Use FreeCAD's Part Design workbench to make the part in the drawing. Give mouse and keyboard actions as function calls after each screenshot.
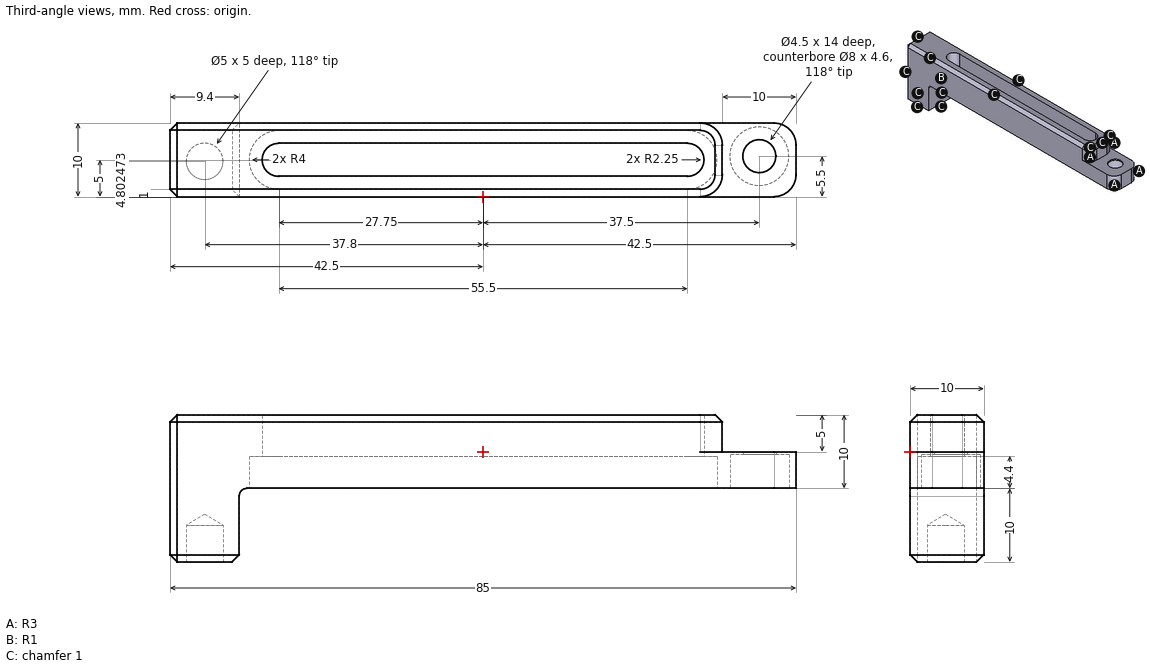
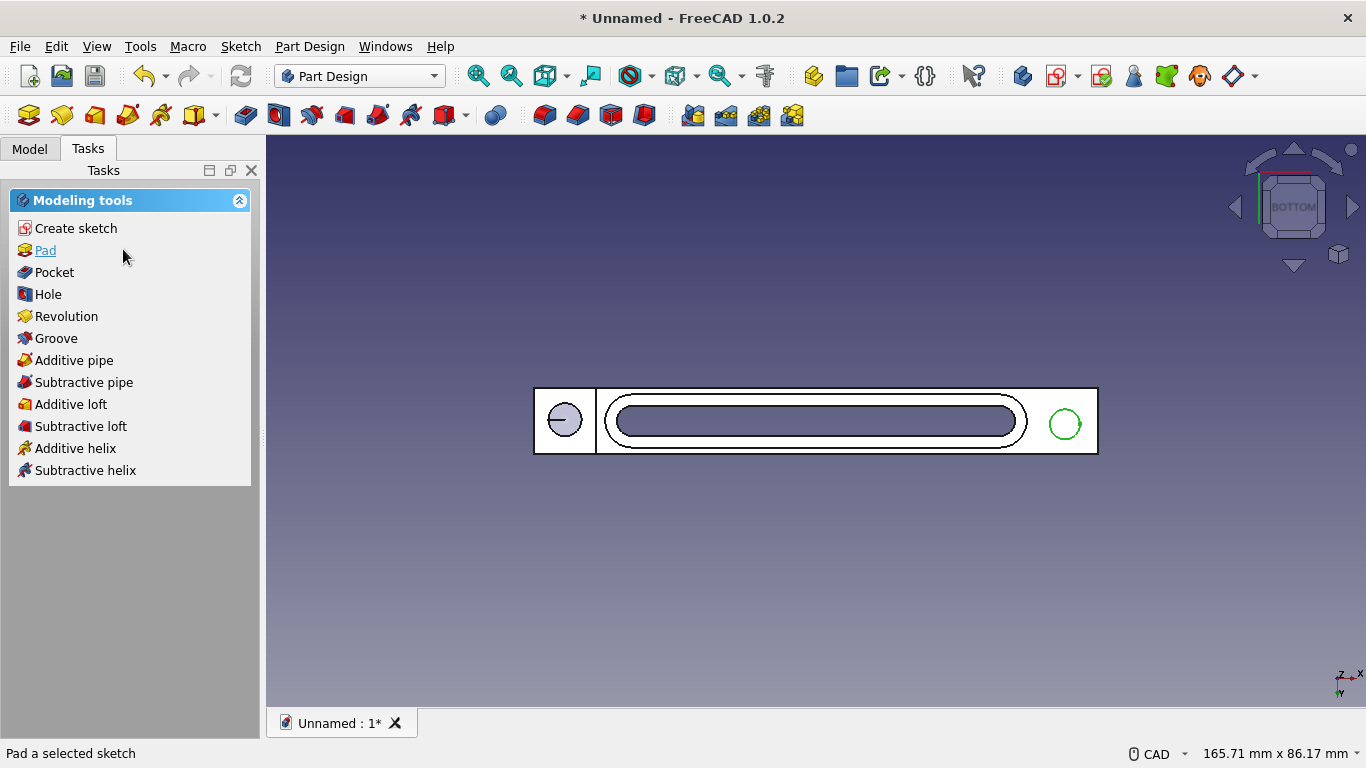
click(279, 116)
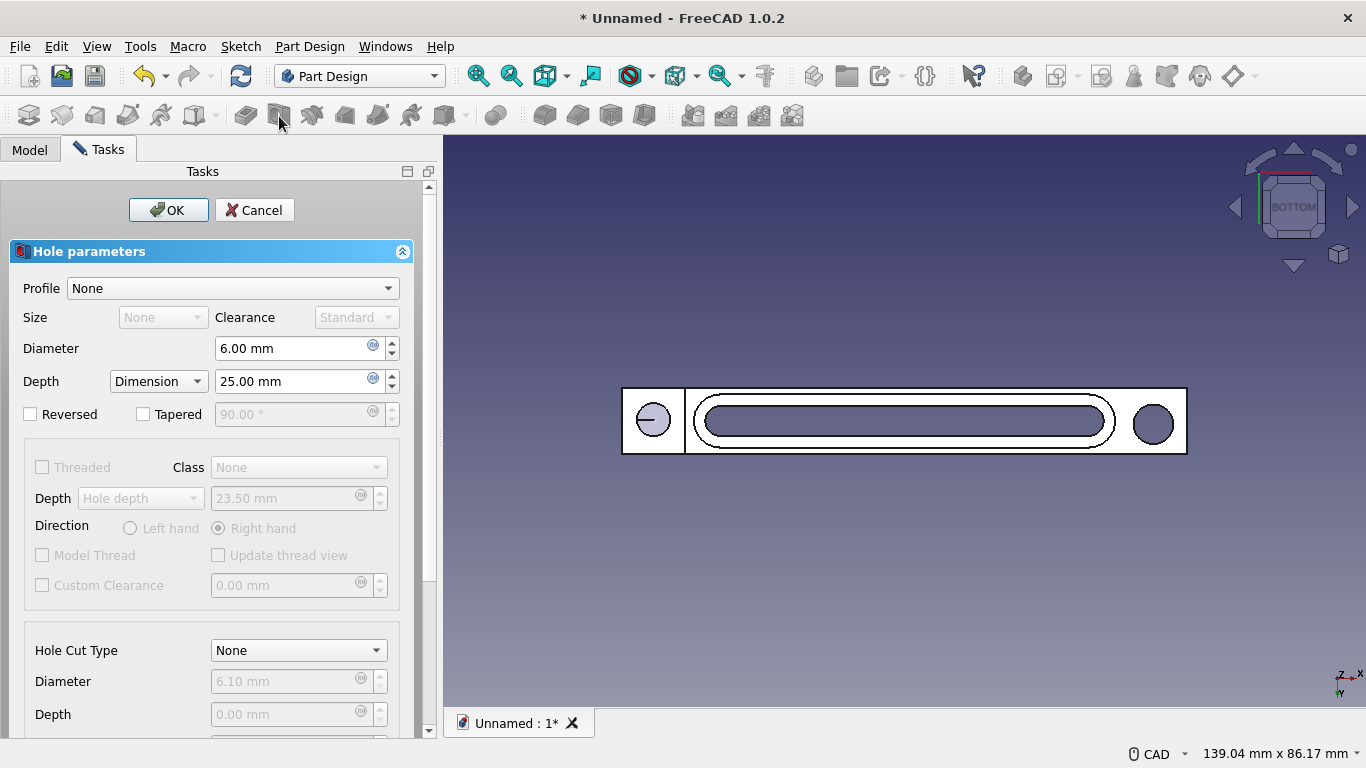
triple_click(300, 348)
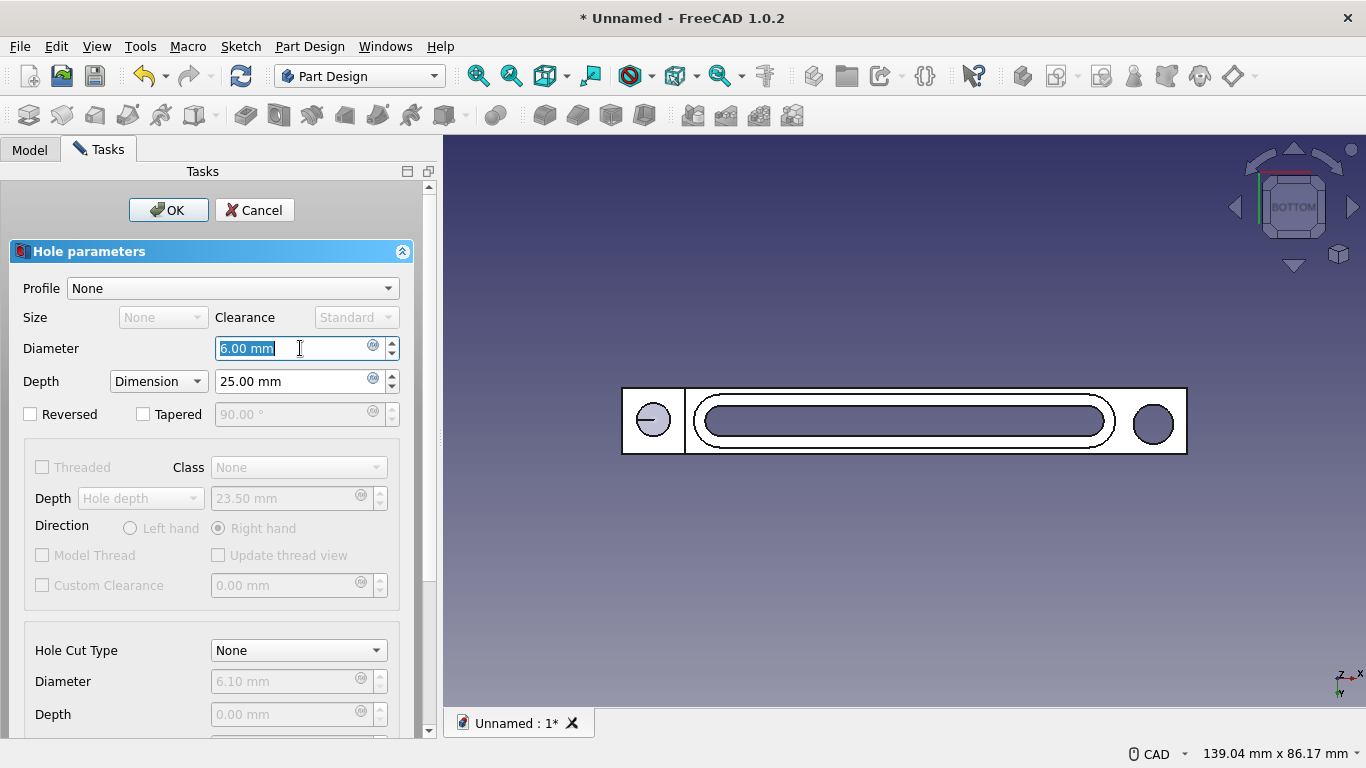
text(4.5)
key(Tab)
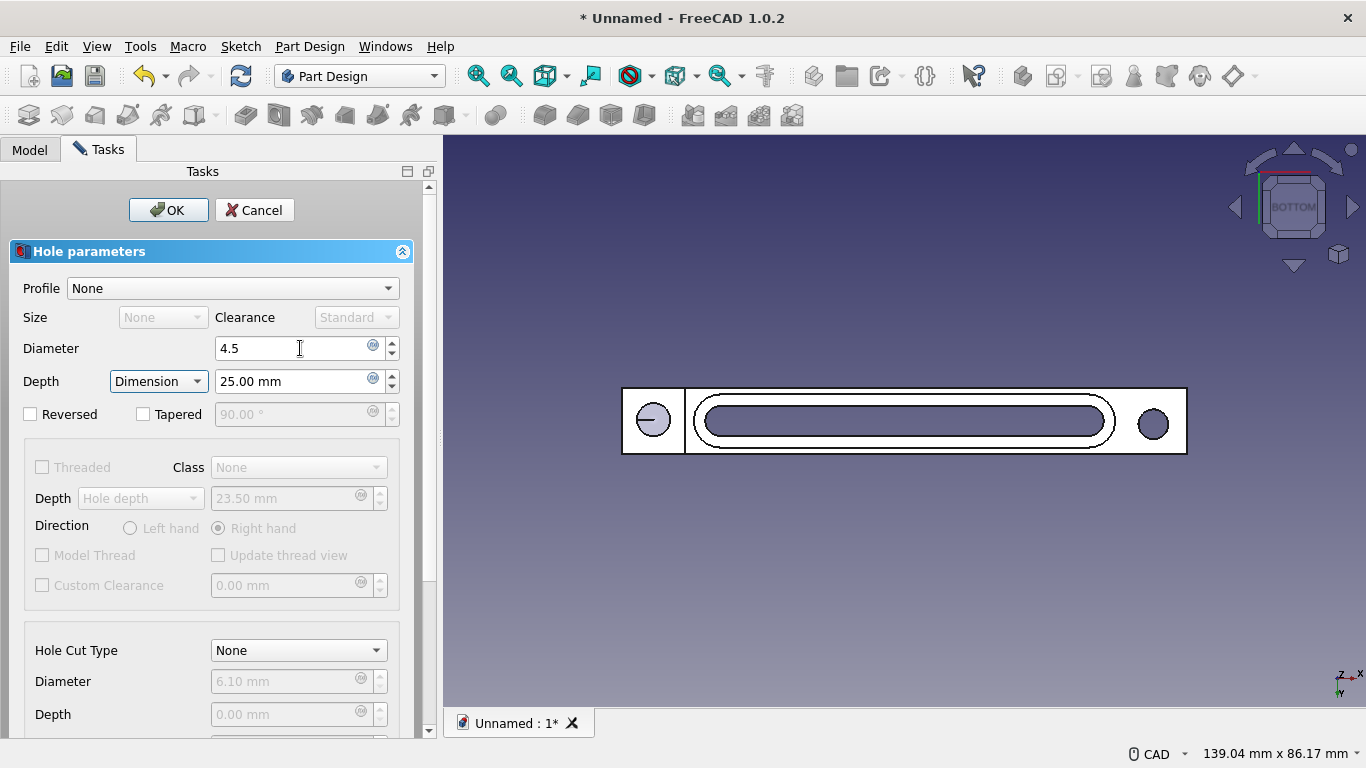
triple_click(300, 382)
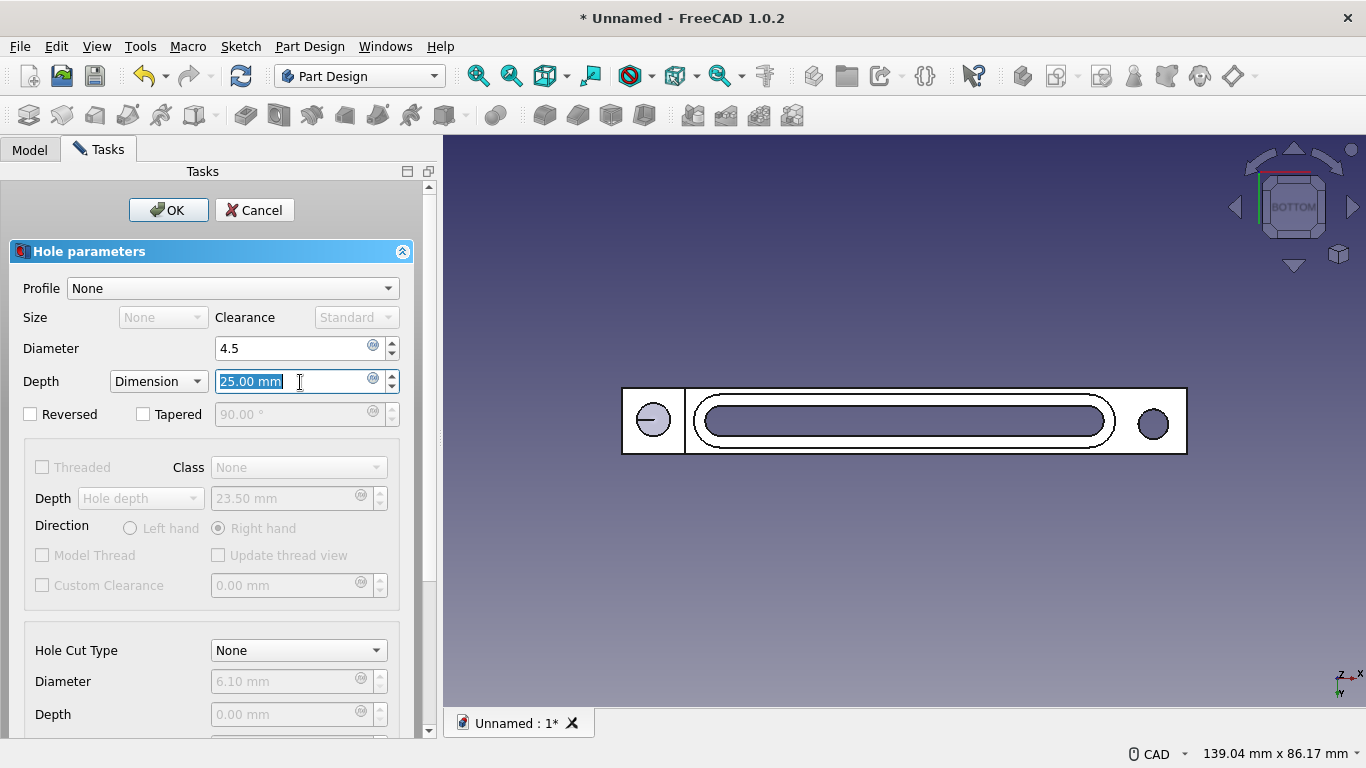
text(14)
key(Tab)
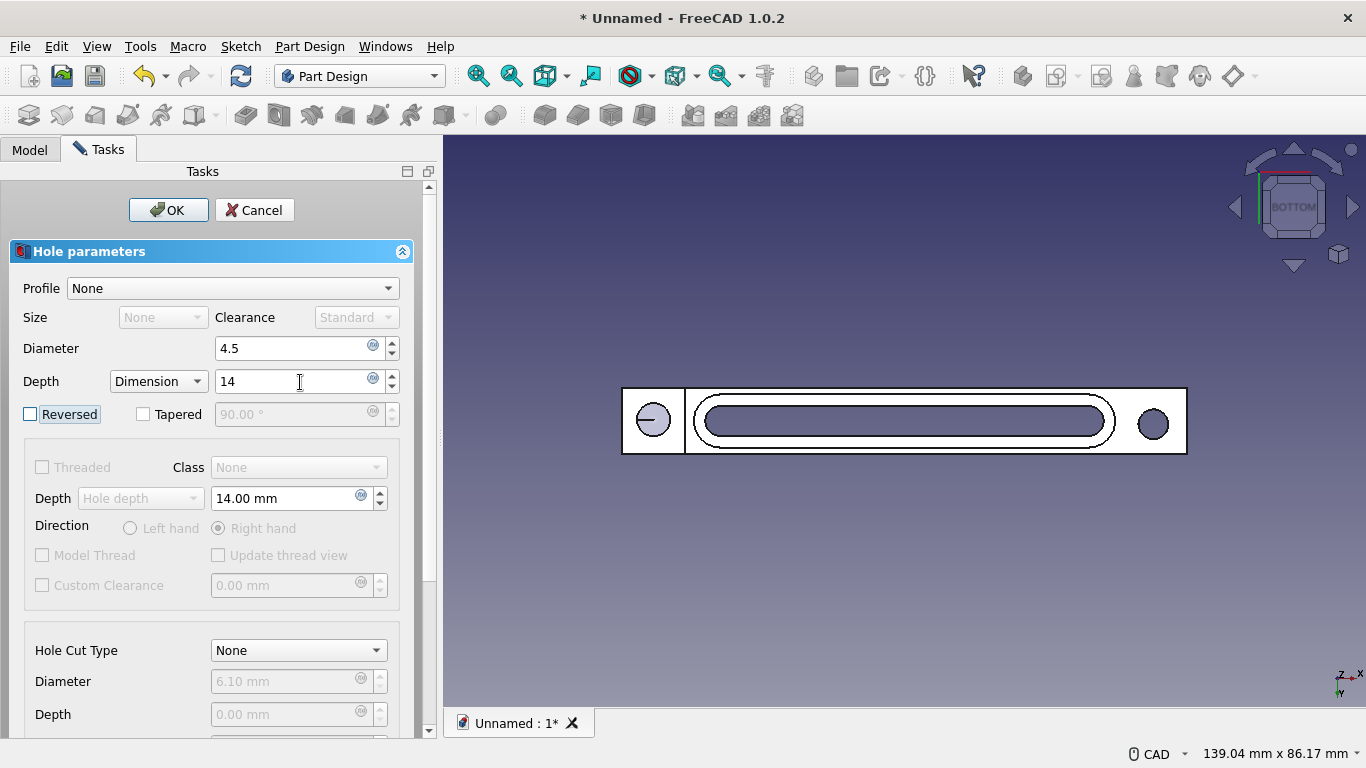
click(300, 650)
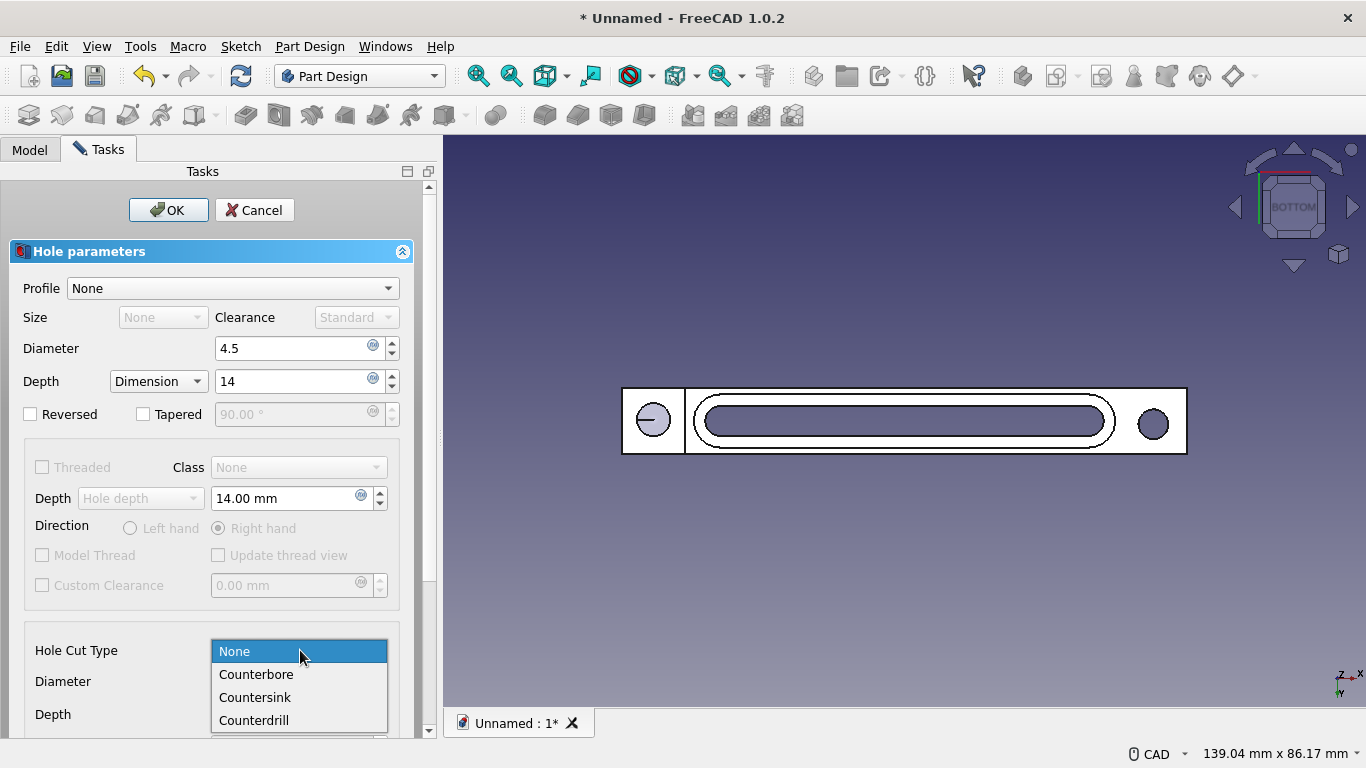
click(298, 674)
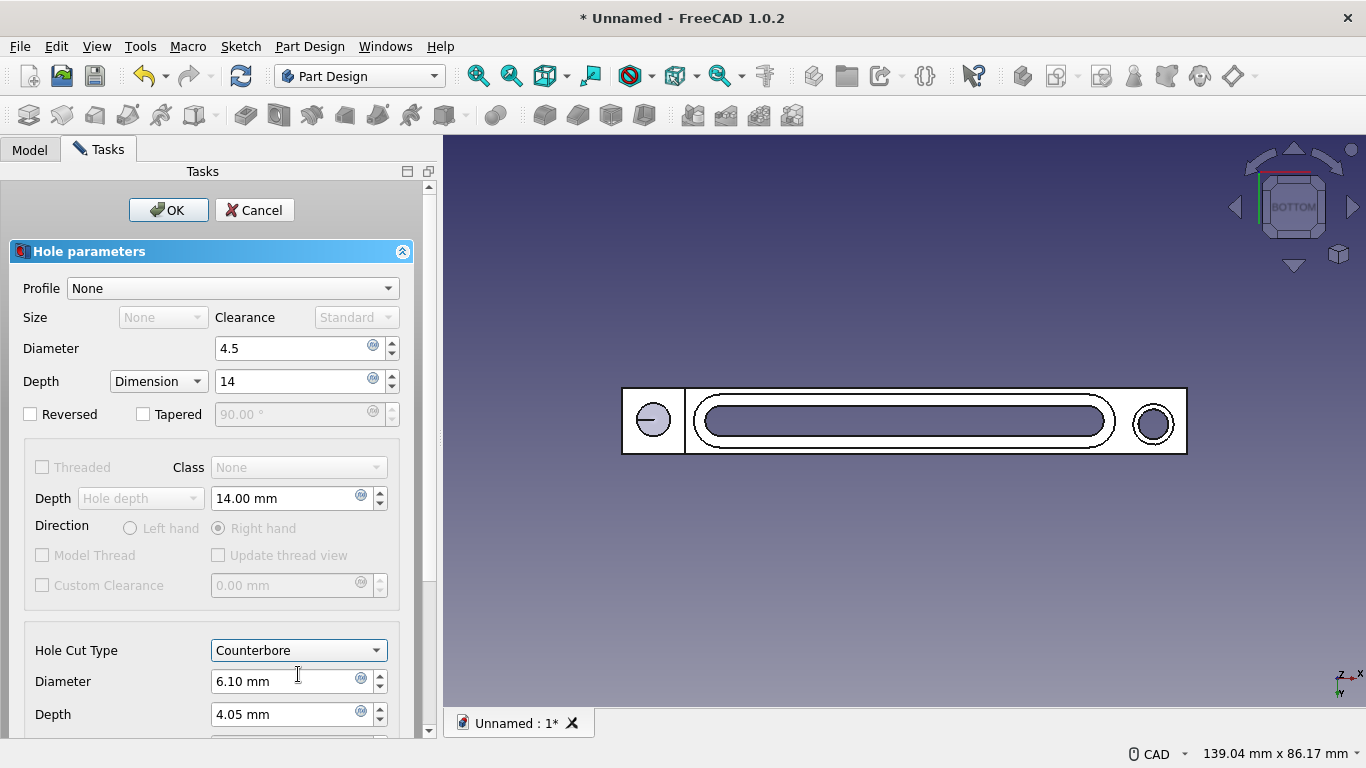
triple_click(292, 682)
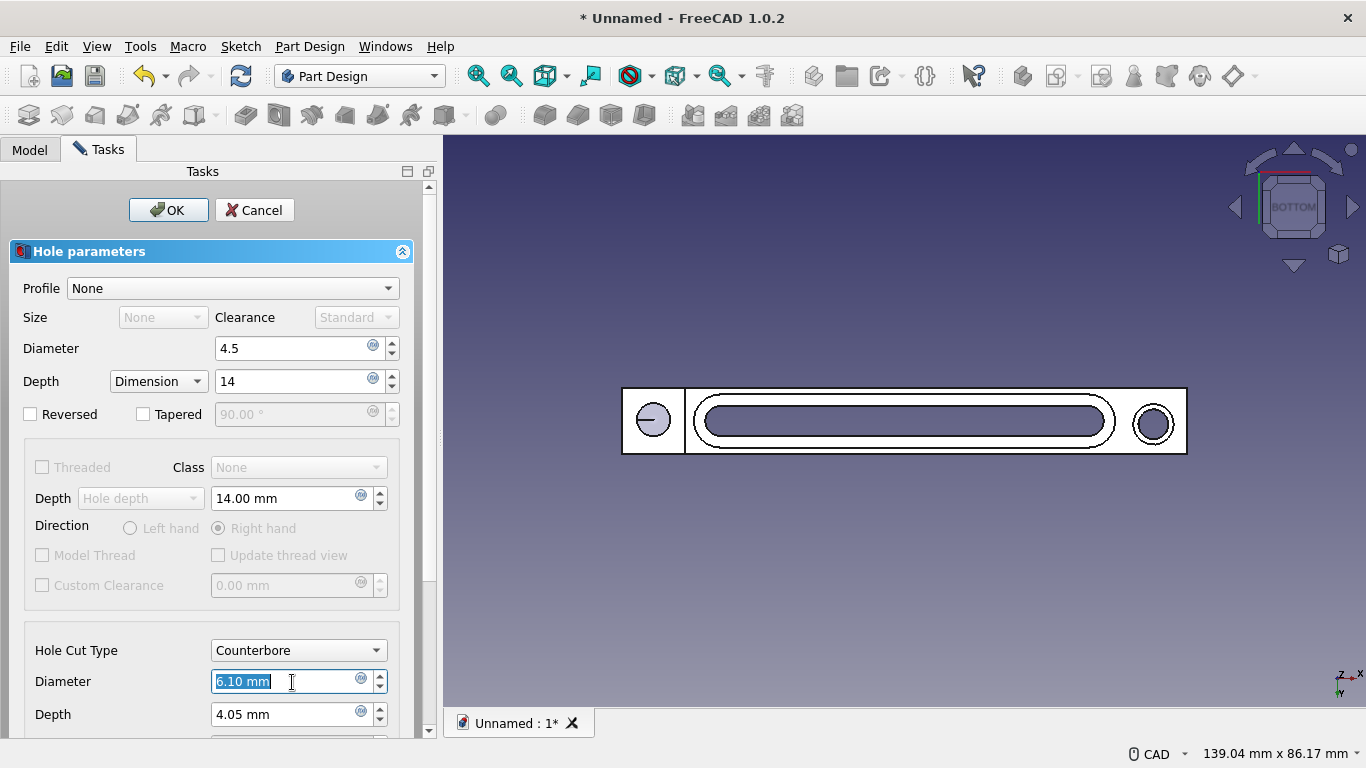
text(8)
key(Tab)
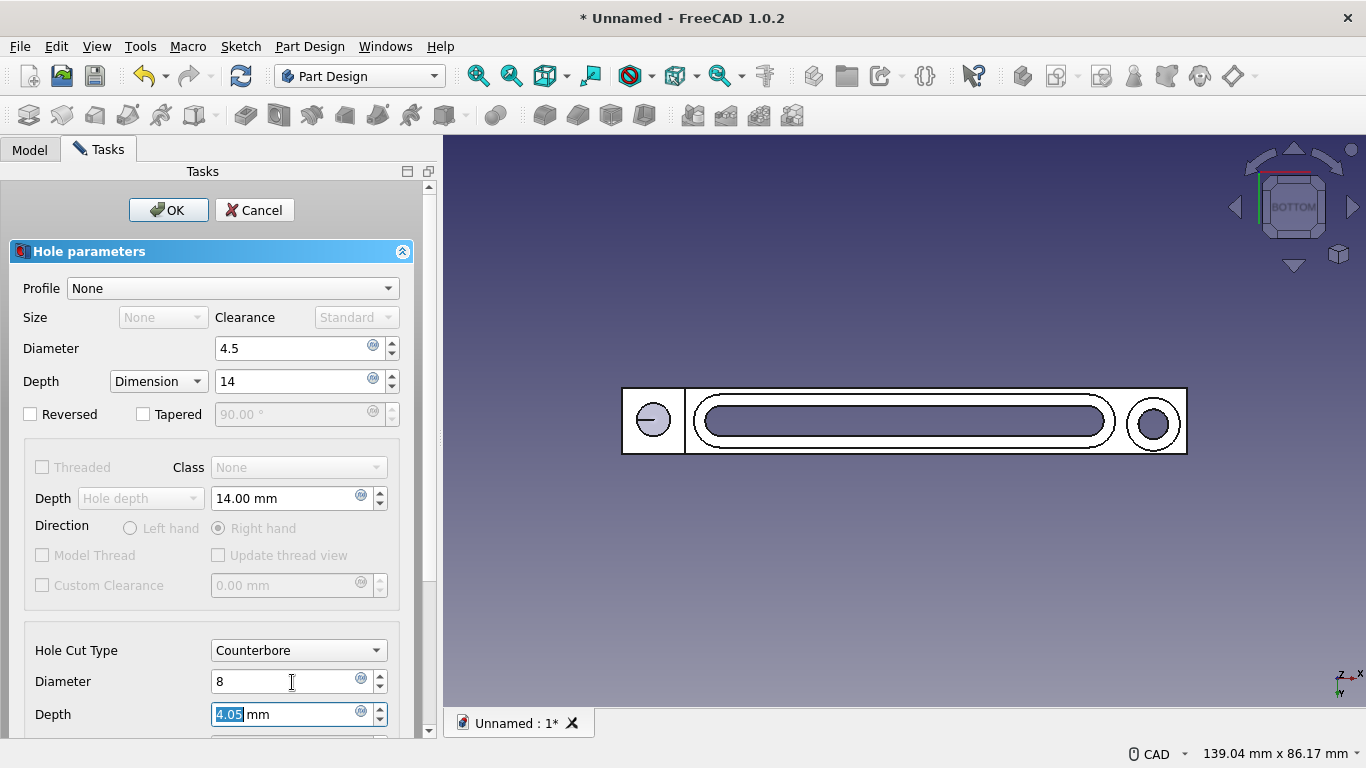
text(4.6)
key(Tab)